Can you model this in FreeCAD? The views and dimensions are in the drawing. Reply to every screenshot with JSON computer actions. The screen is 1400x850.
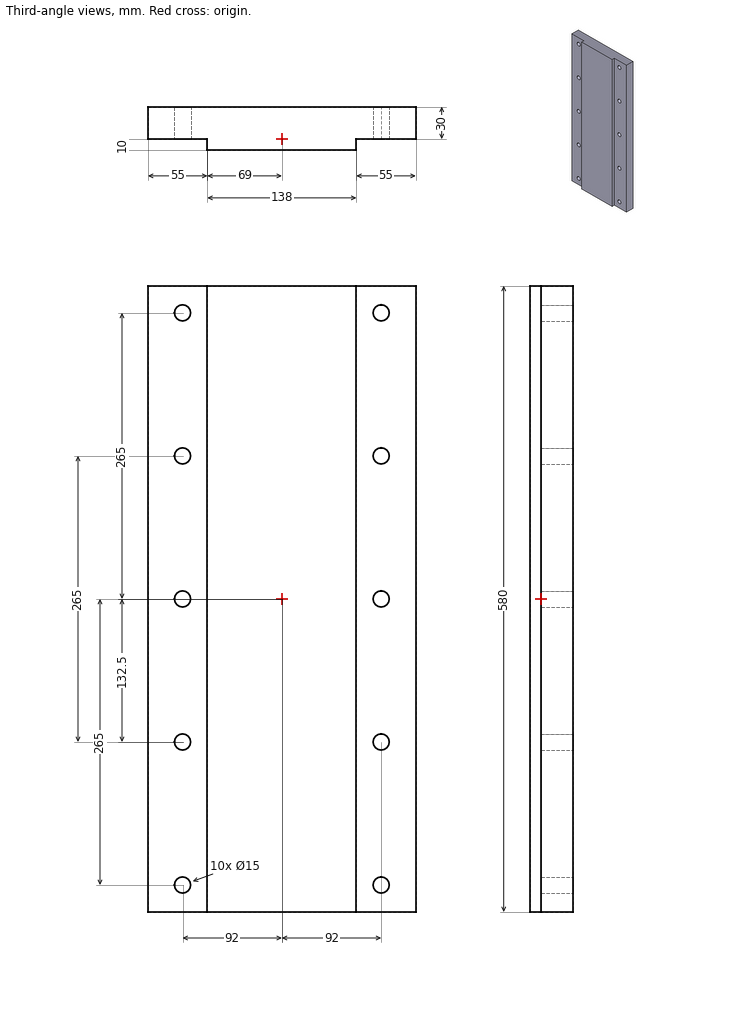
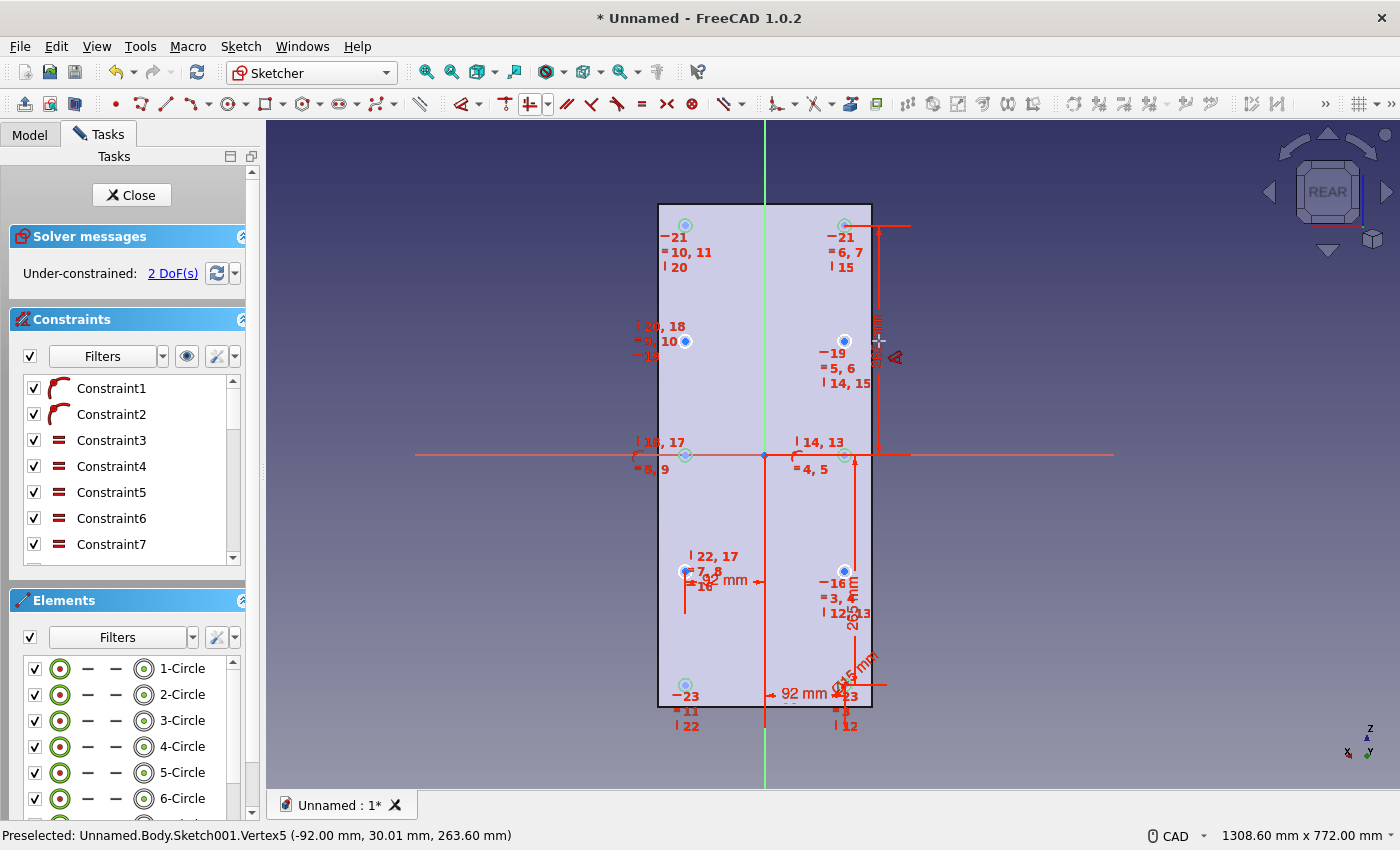
{"action": "left_click", "coordinate": [845, 572]}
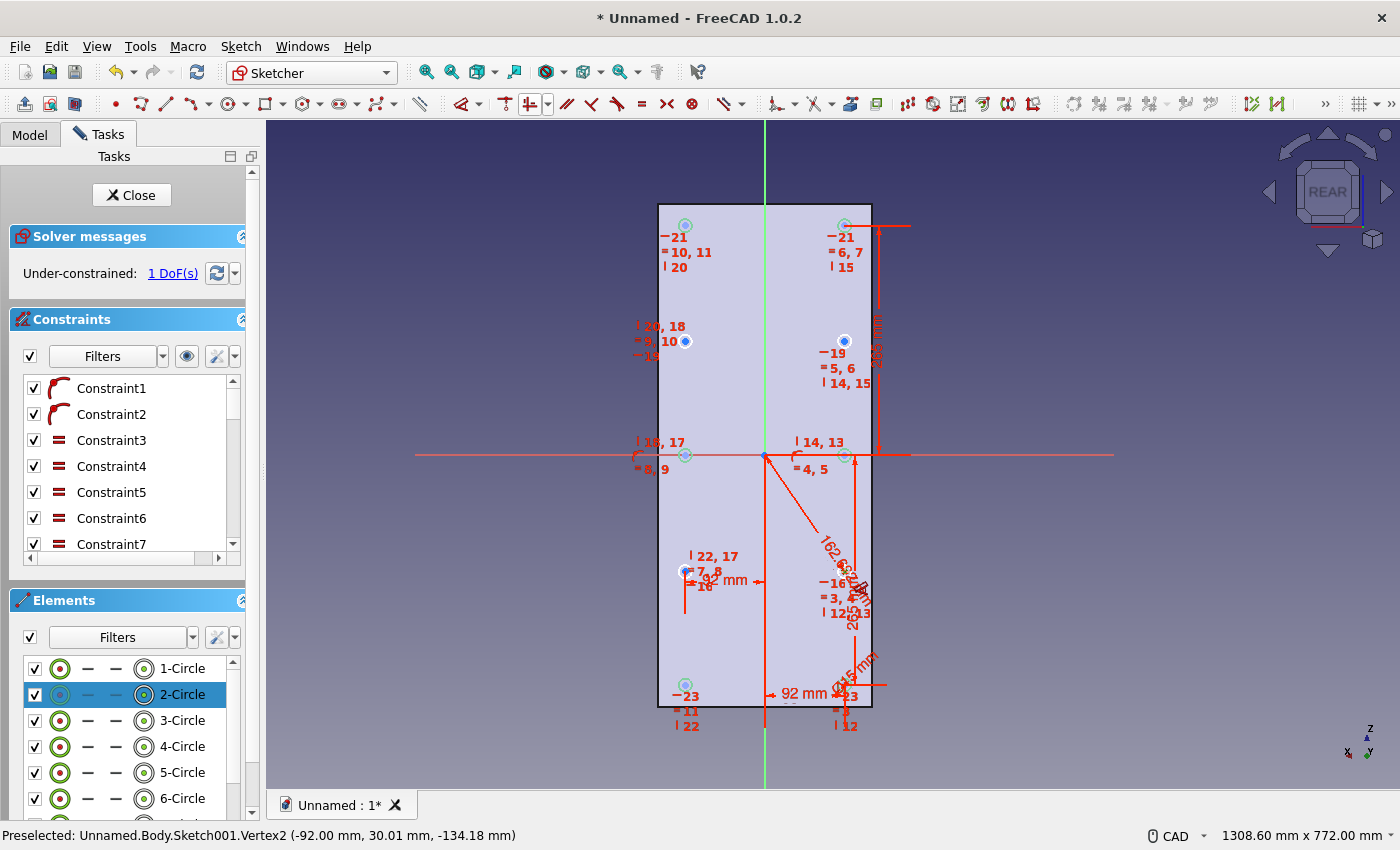
{"action": "left_click", "coordinate": [845, 341]}
{"action": "left_click", "coordinate": [879, 404]}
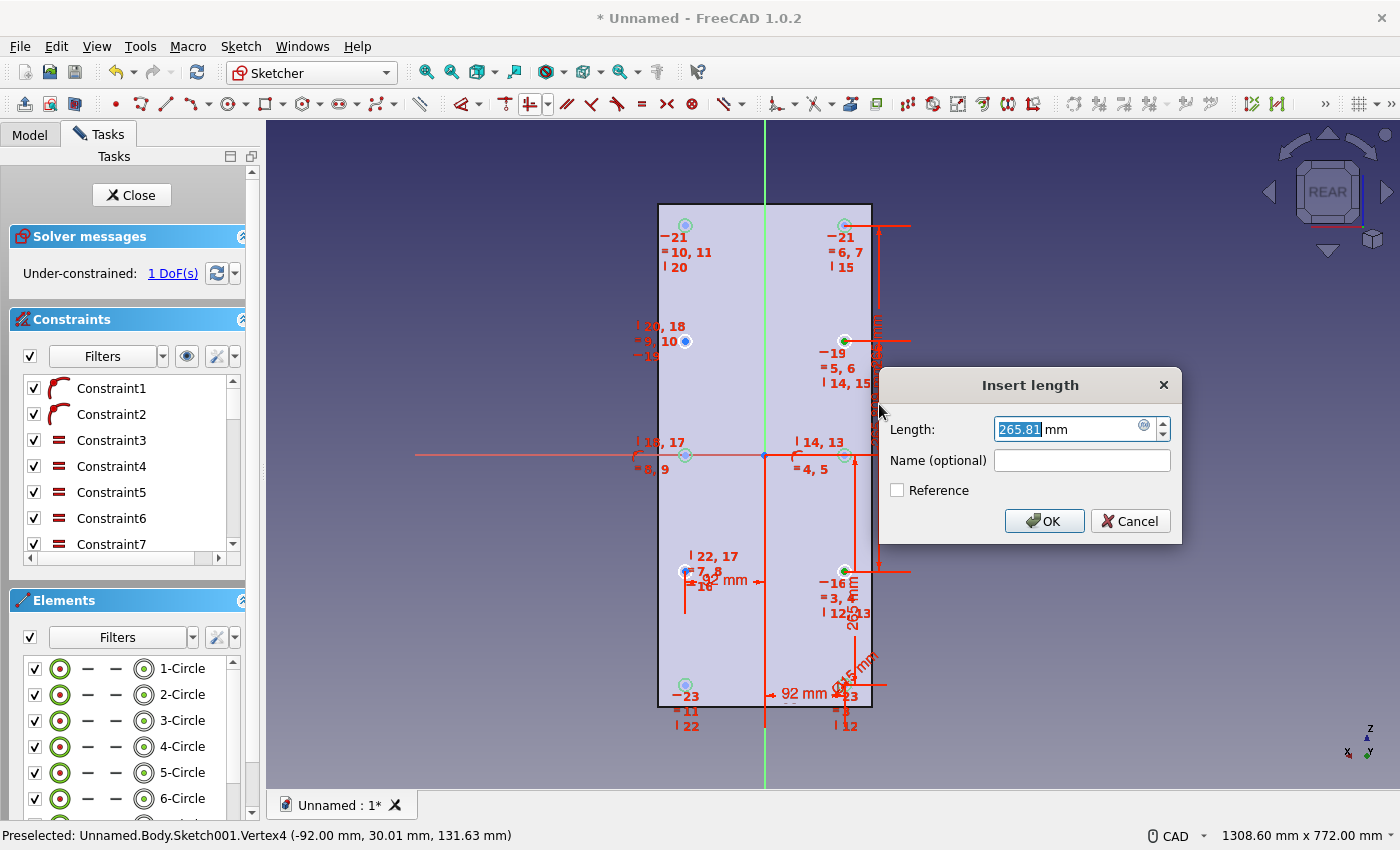
{"action": "type", "text": "265"}
{"action": "key", "text": "Return"}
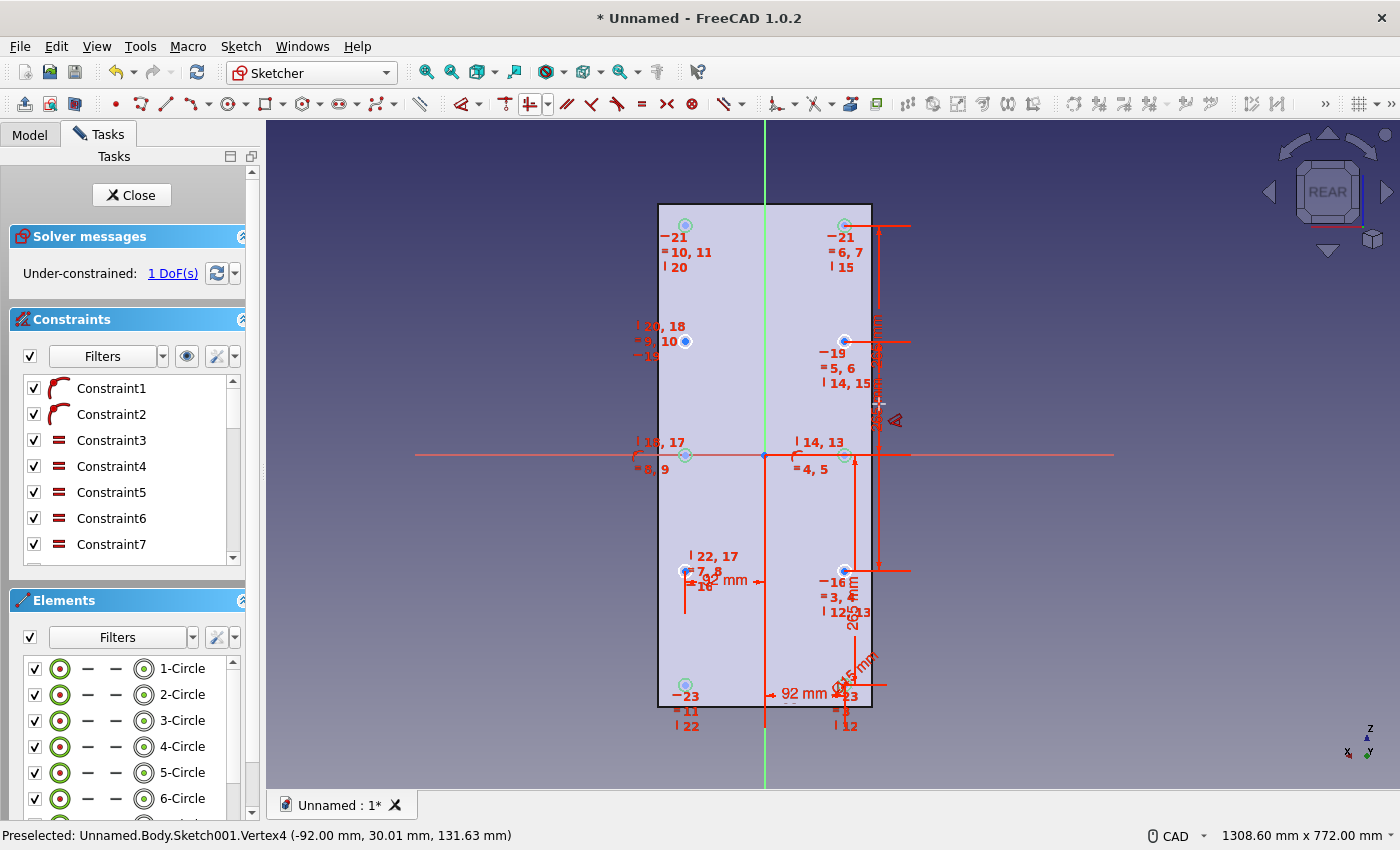
{"action": "left_click", "coordinate": [845, 571]}
{"action": "left_click", "coordinate": [879, 513]}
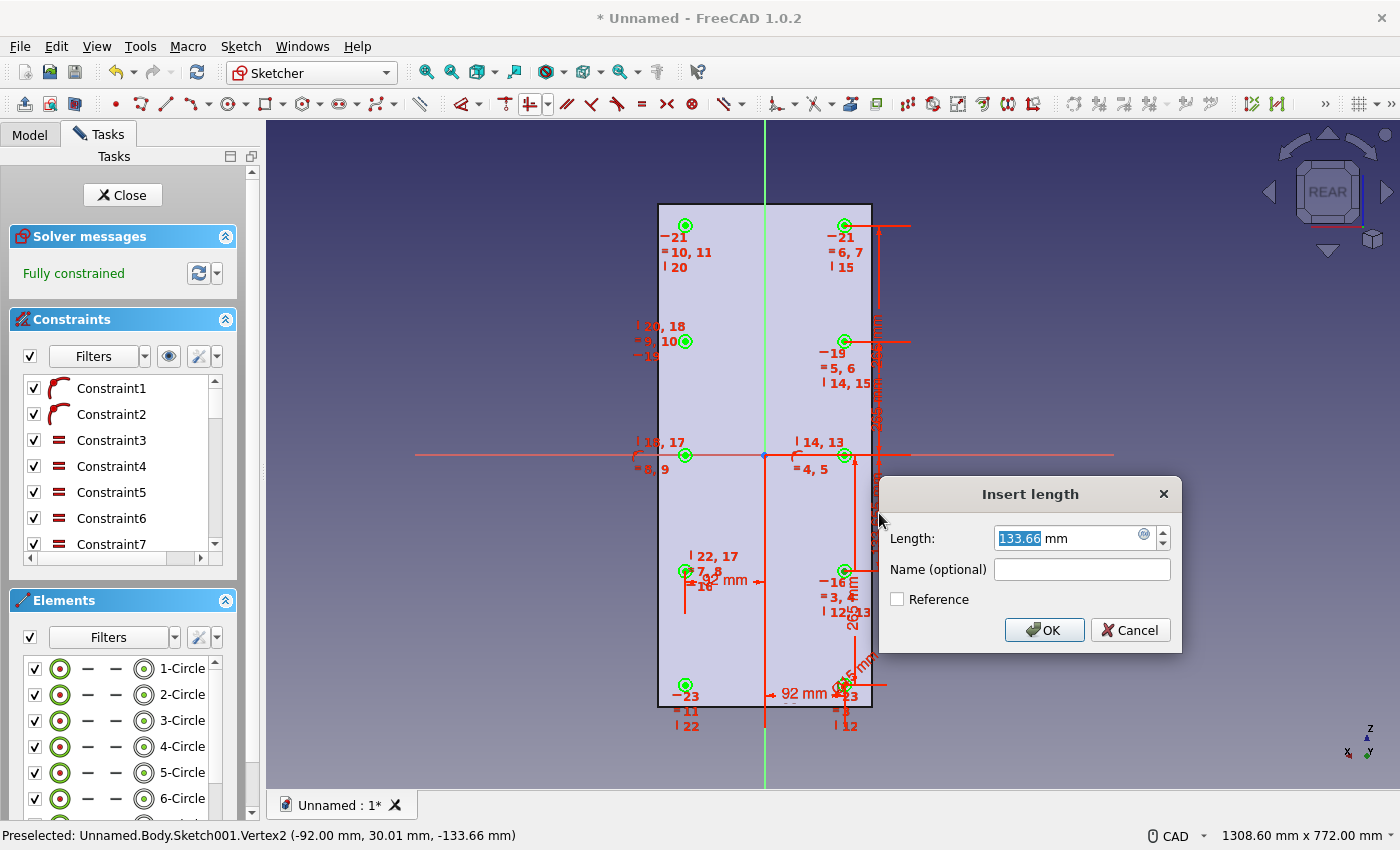
{"action": "type", "text": "132.5"}
{"action": "key", "text": "Return"}
{"action": "key", "text": "Escape"}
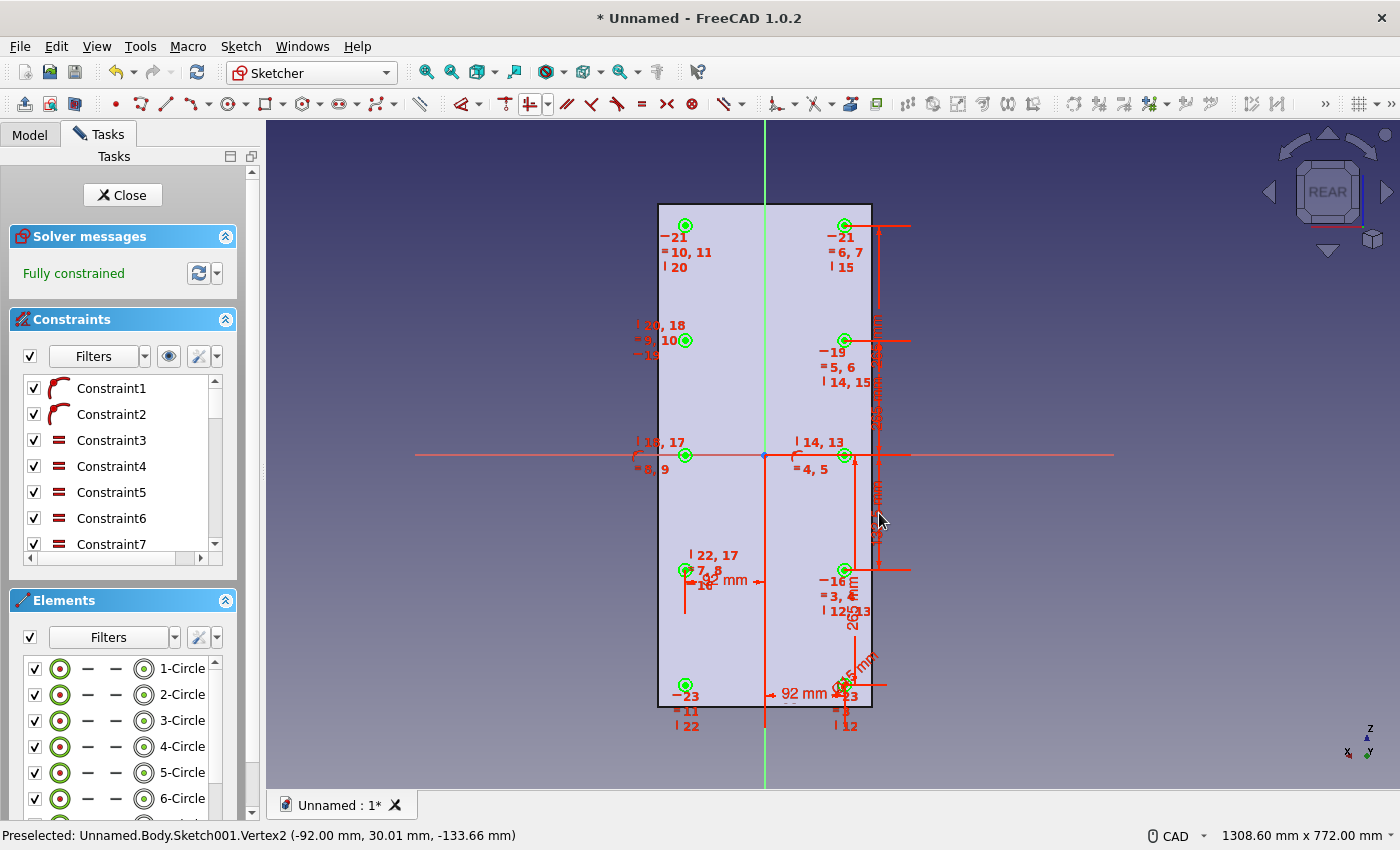
{"action": "left_click", "coordinate": [123, 195]}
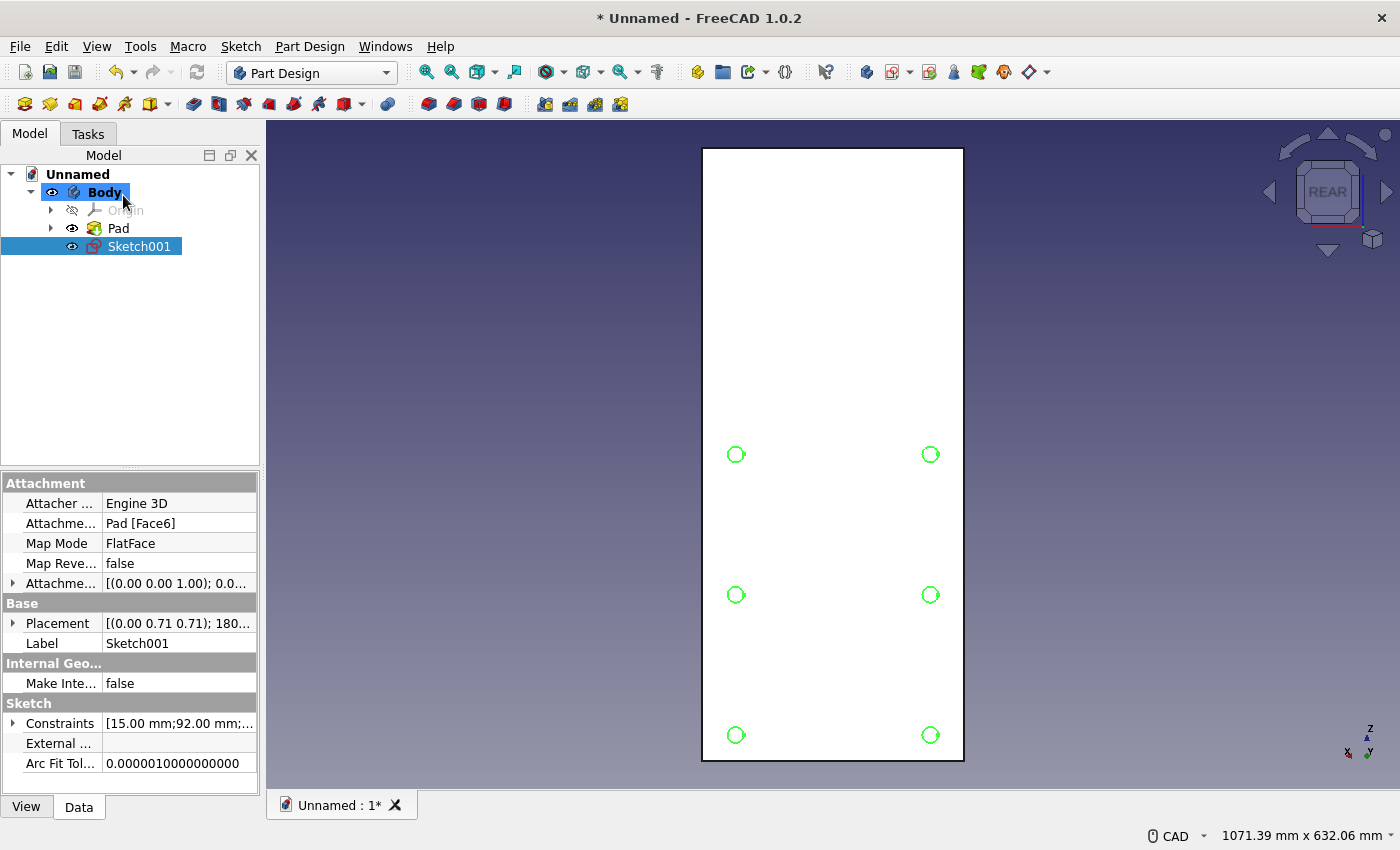
{"action": "left_click", "coordinate": [194, 104]}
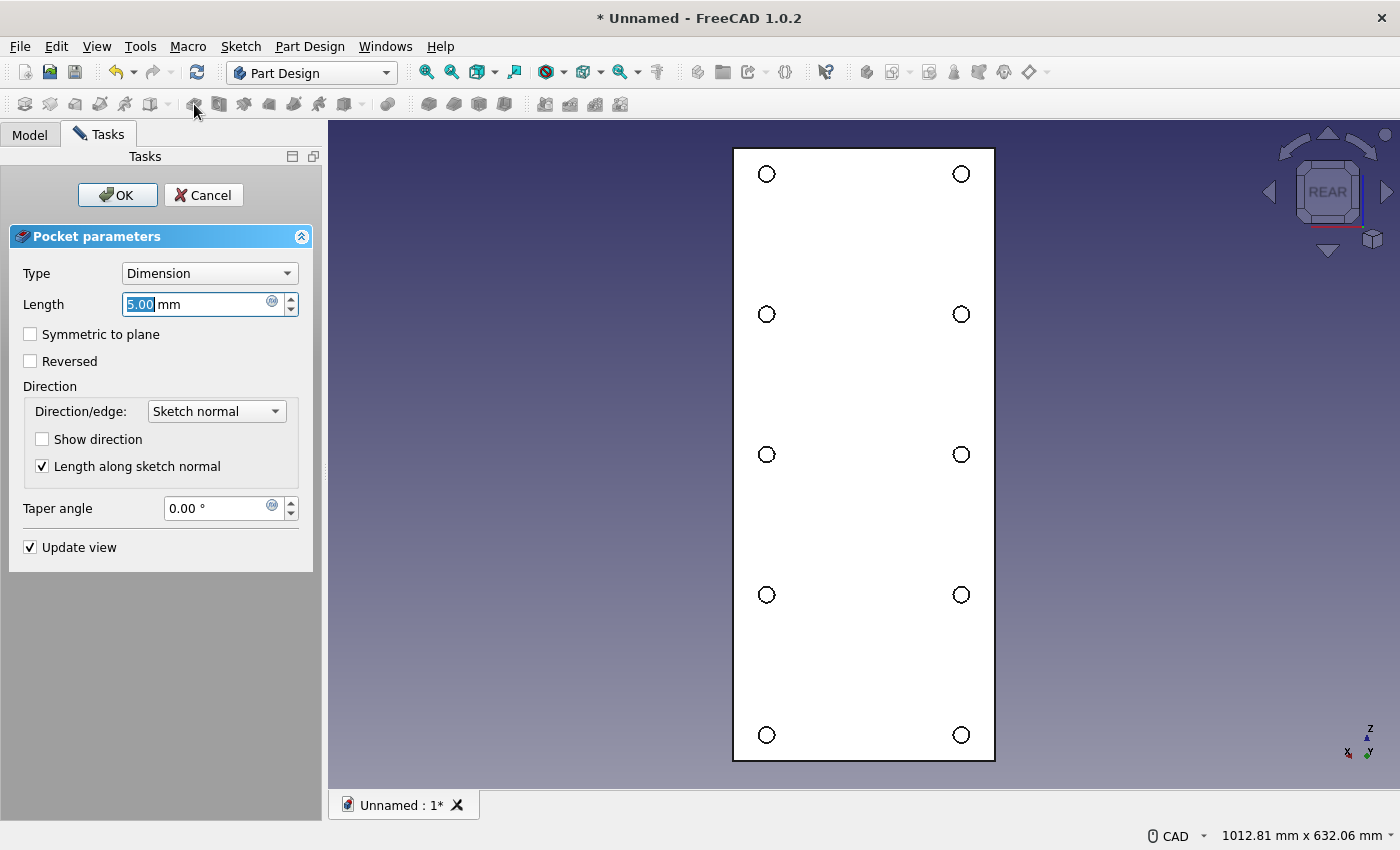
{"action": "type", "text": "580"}
{"action": "key", "text": "Tab"}